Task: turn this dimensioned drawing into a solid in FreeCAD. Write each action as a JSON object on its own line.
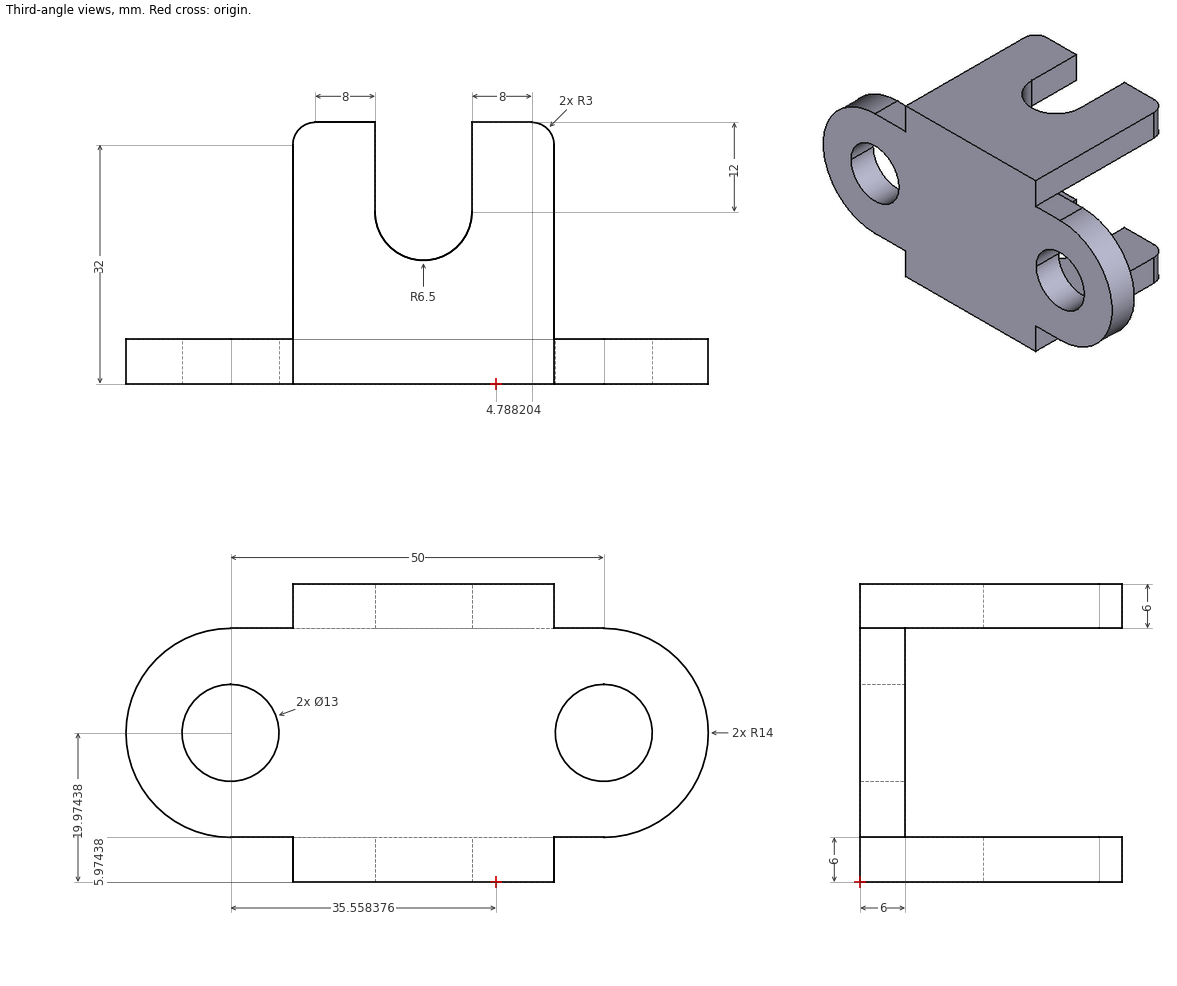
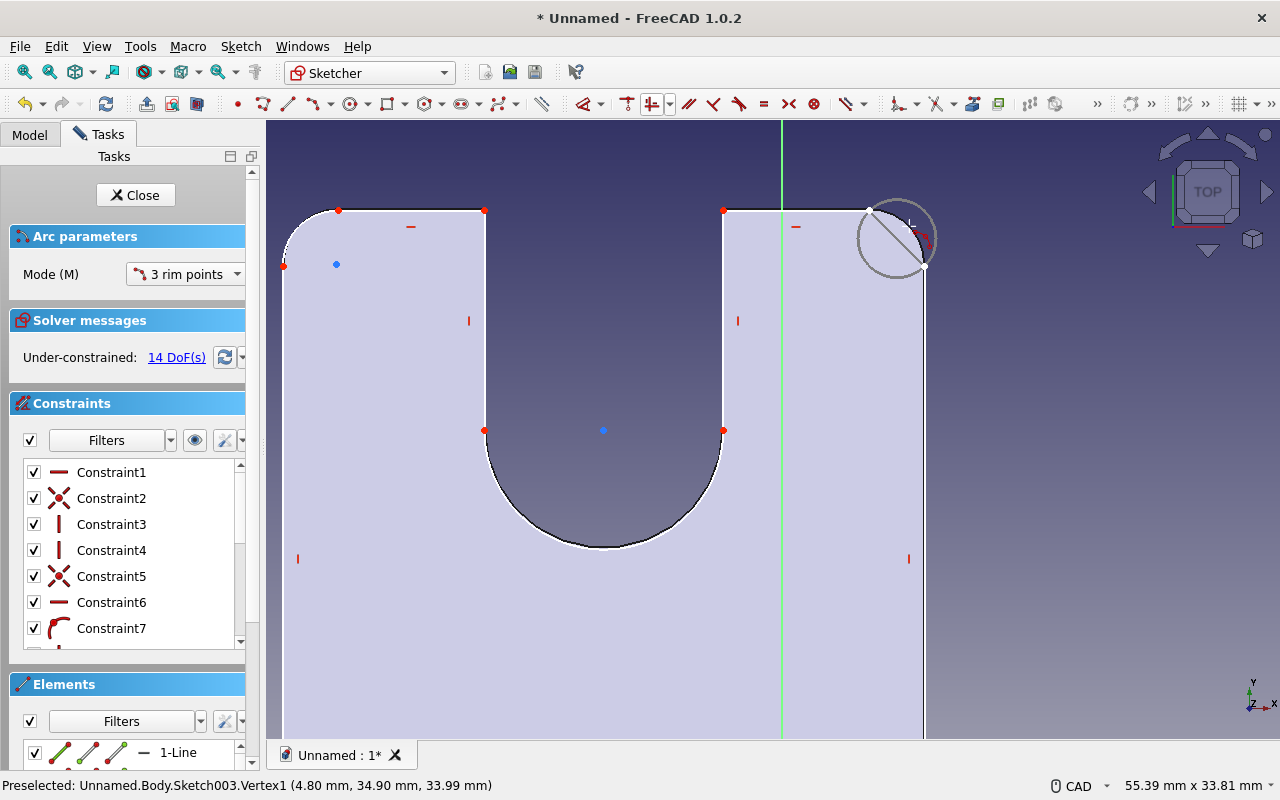
{"action": "left_click", "coordinate": [908, 225]}
{"action": "key", "text": "Escape"}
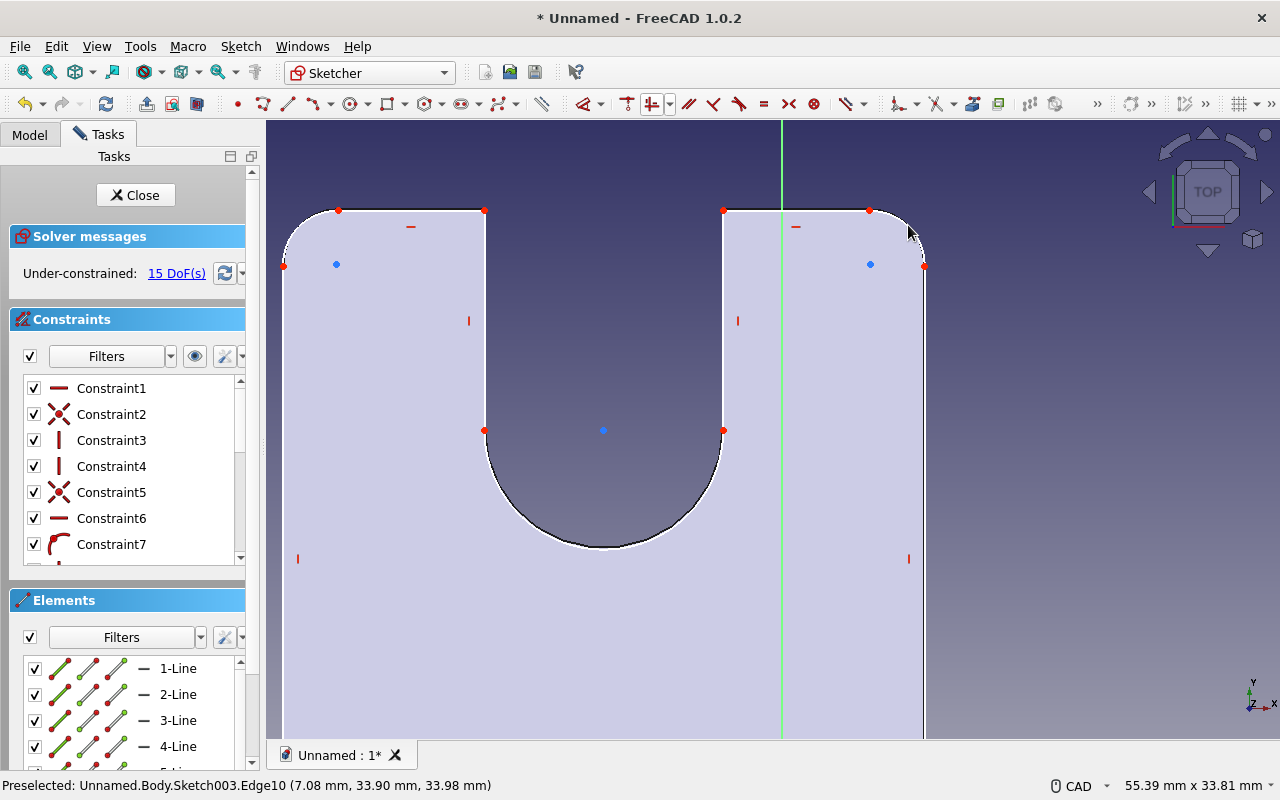
{"action": "left_click", "coordinate": [826, 211]}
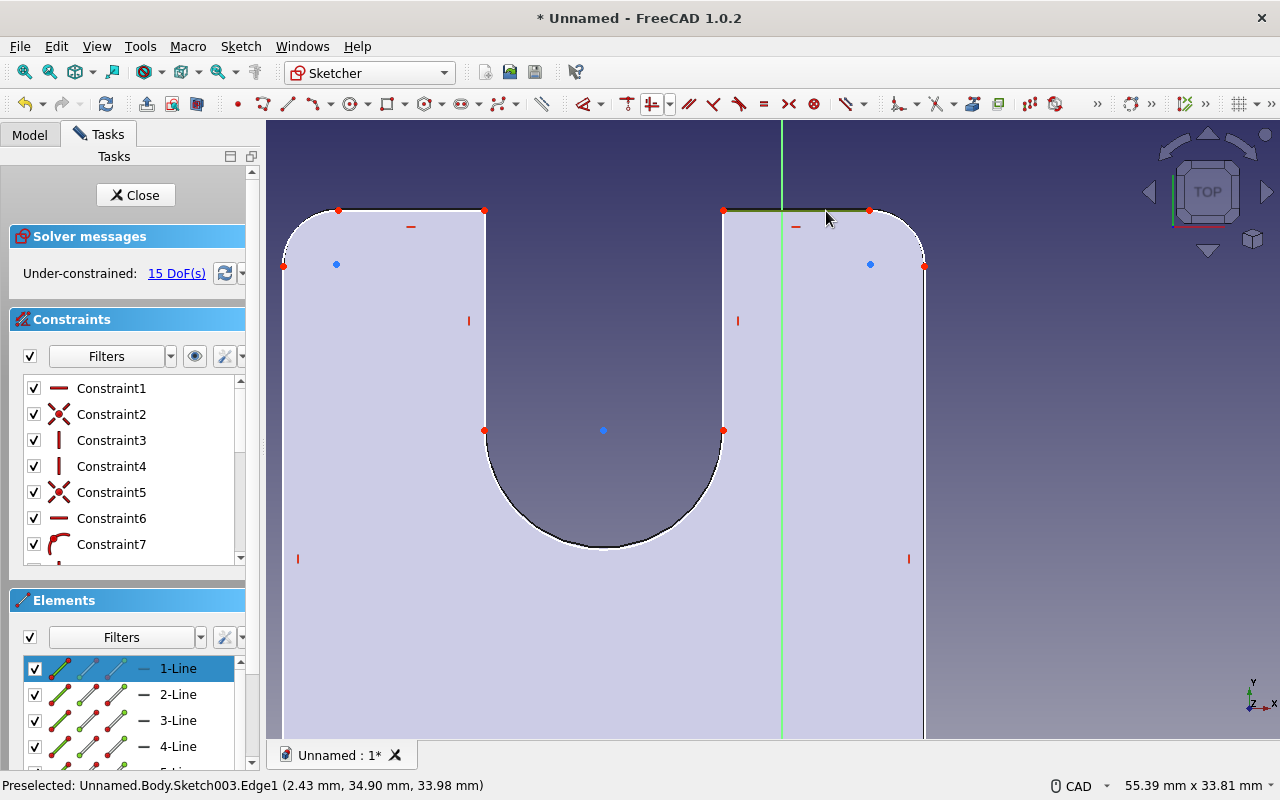
{"action": "left_click", "coordinate": [919, 241]}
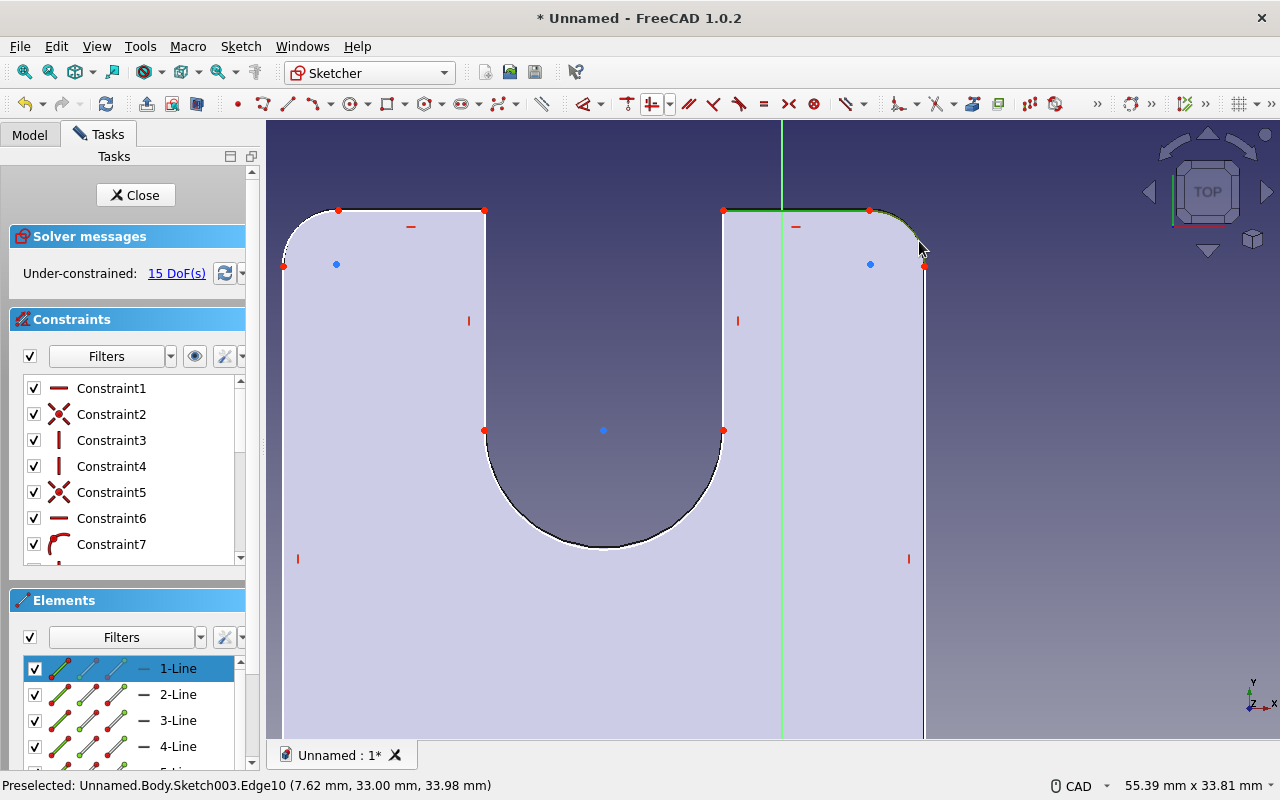
{"action": "left_click", "coordinate": [739, 104]}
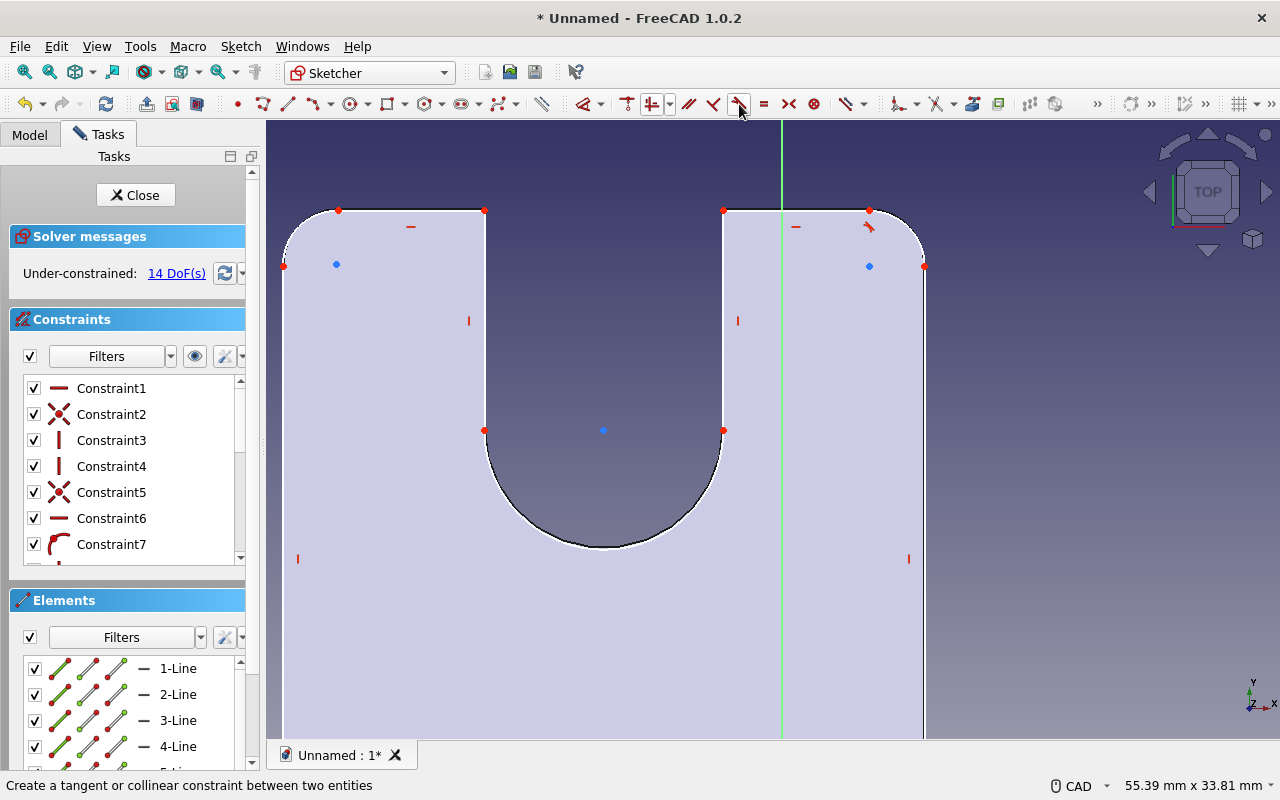
{"action": "left_click", "coordinate": [723, 277]}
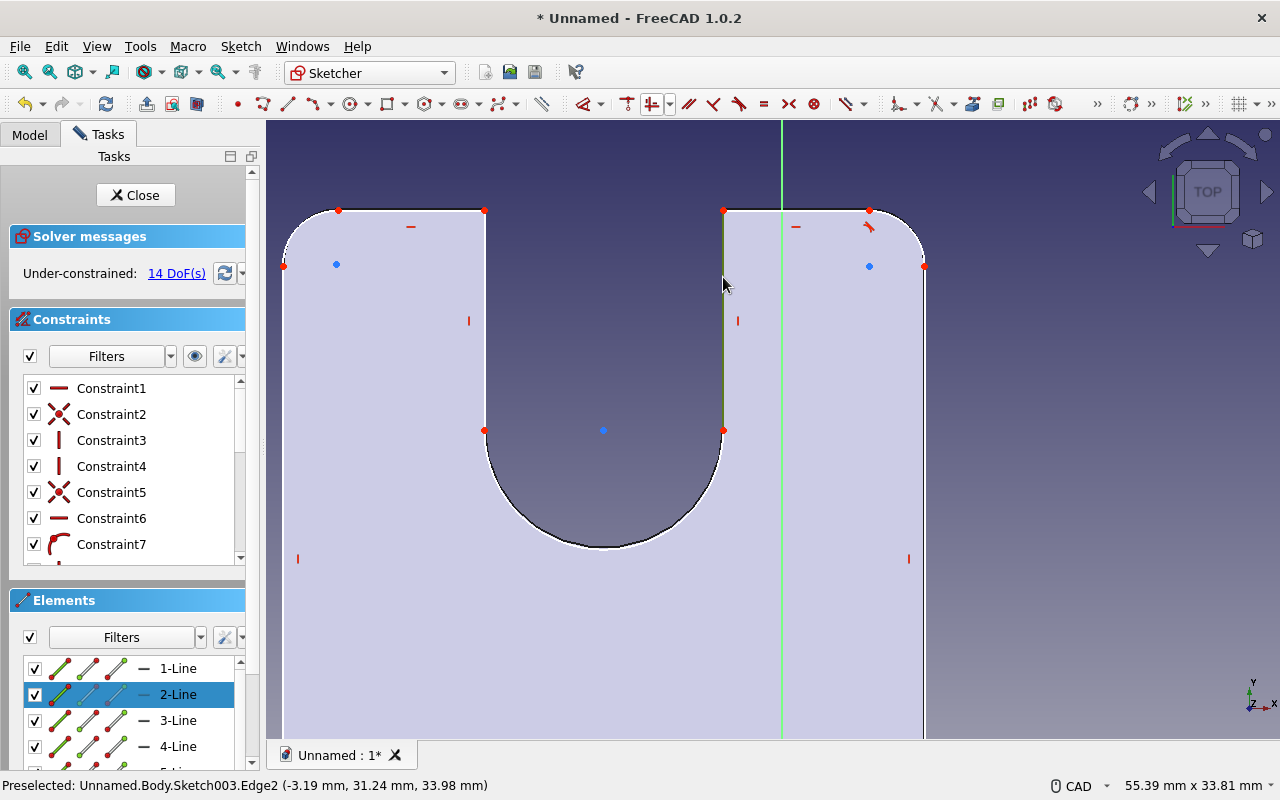
{"action": "left_click", "coordinate": [534, 527]}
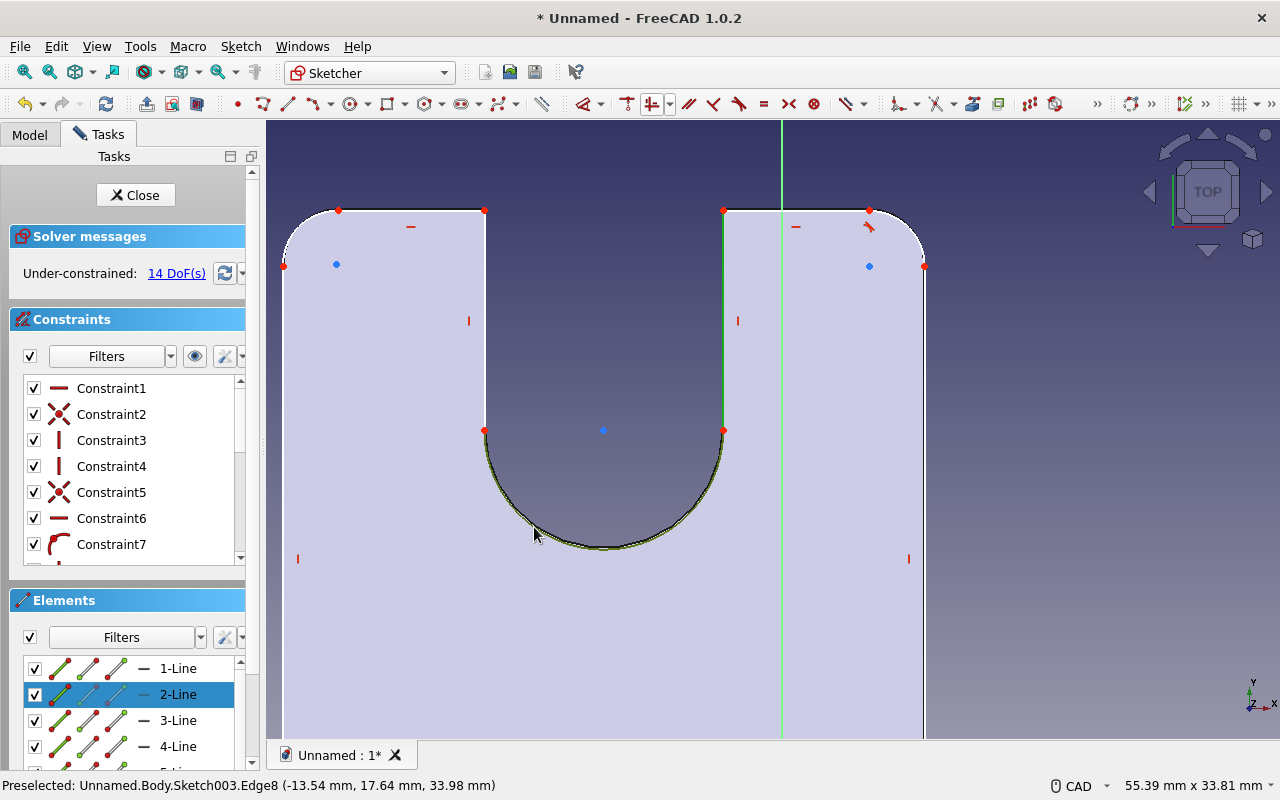
{"action": "left_click", "coordinate": [739, 104]}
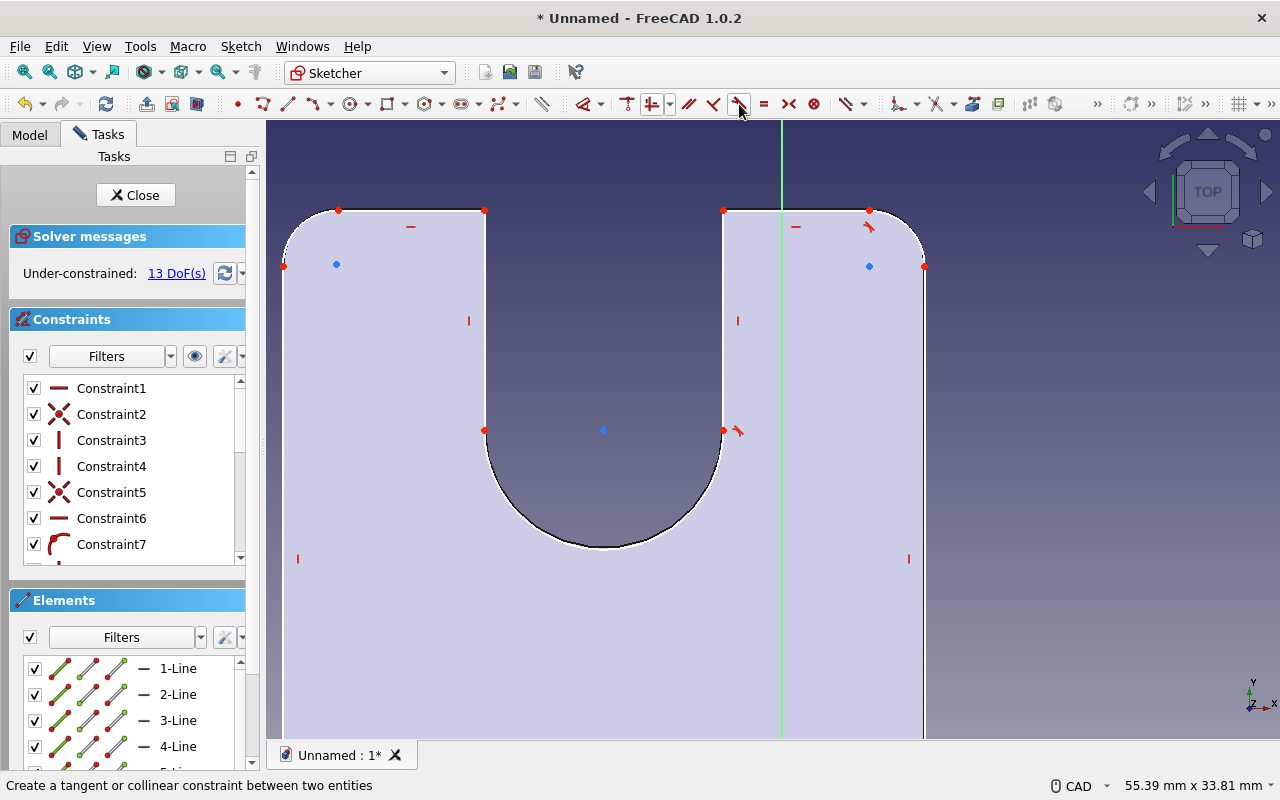
{"action": "left_click", "coordinate": [485, 365]}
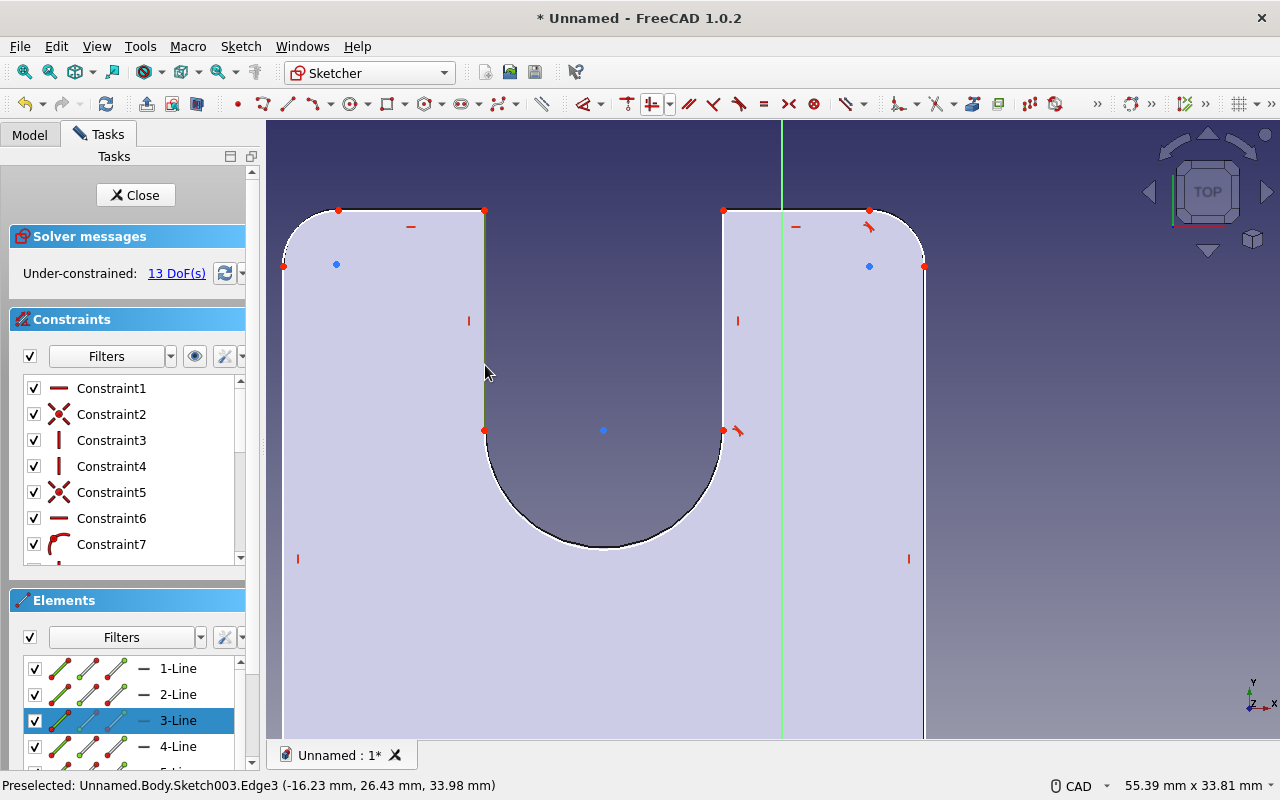
{"action": "left_click", "coordinate": [534, 527]}